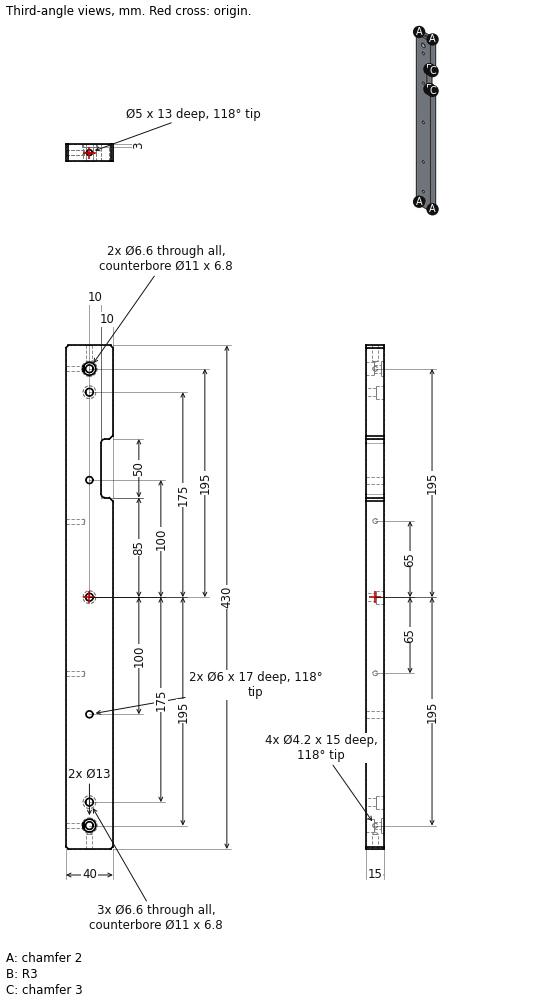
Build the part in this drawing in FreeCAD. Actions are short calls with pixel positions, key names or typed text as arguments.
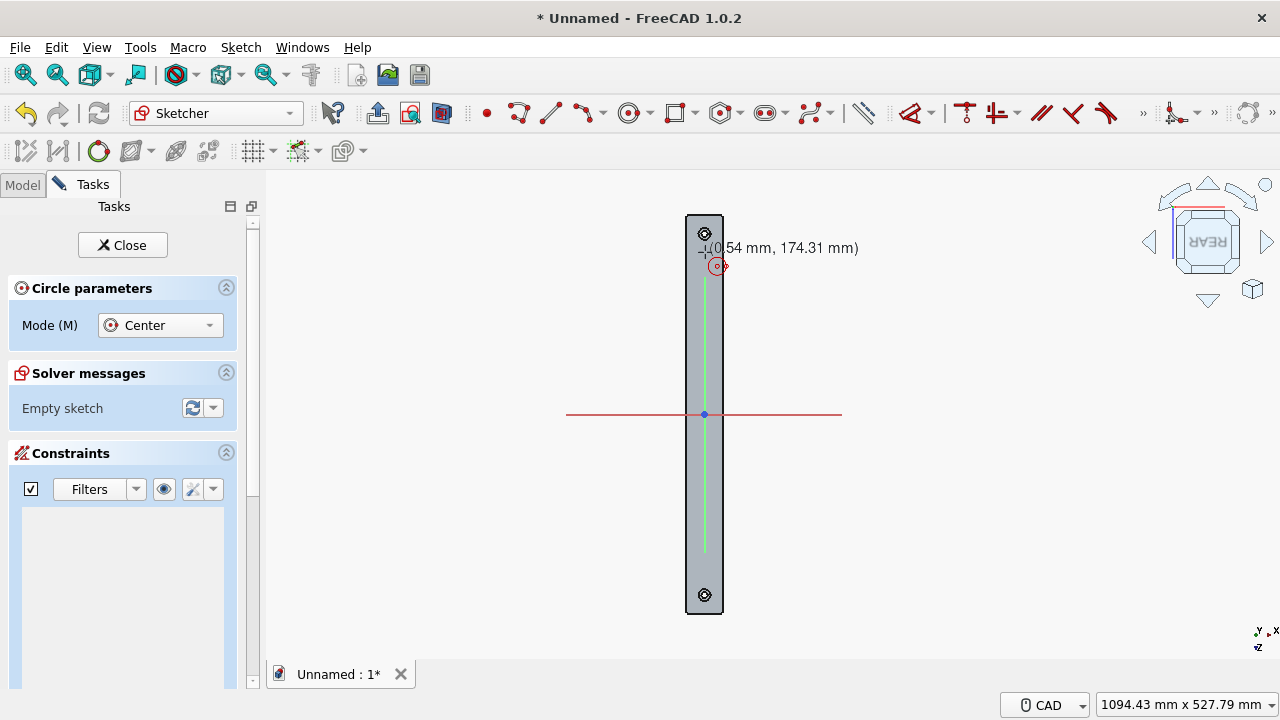
click(705, 252)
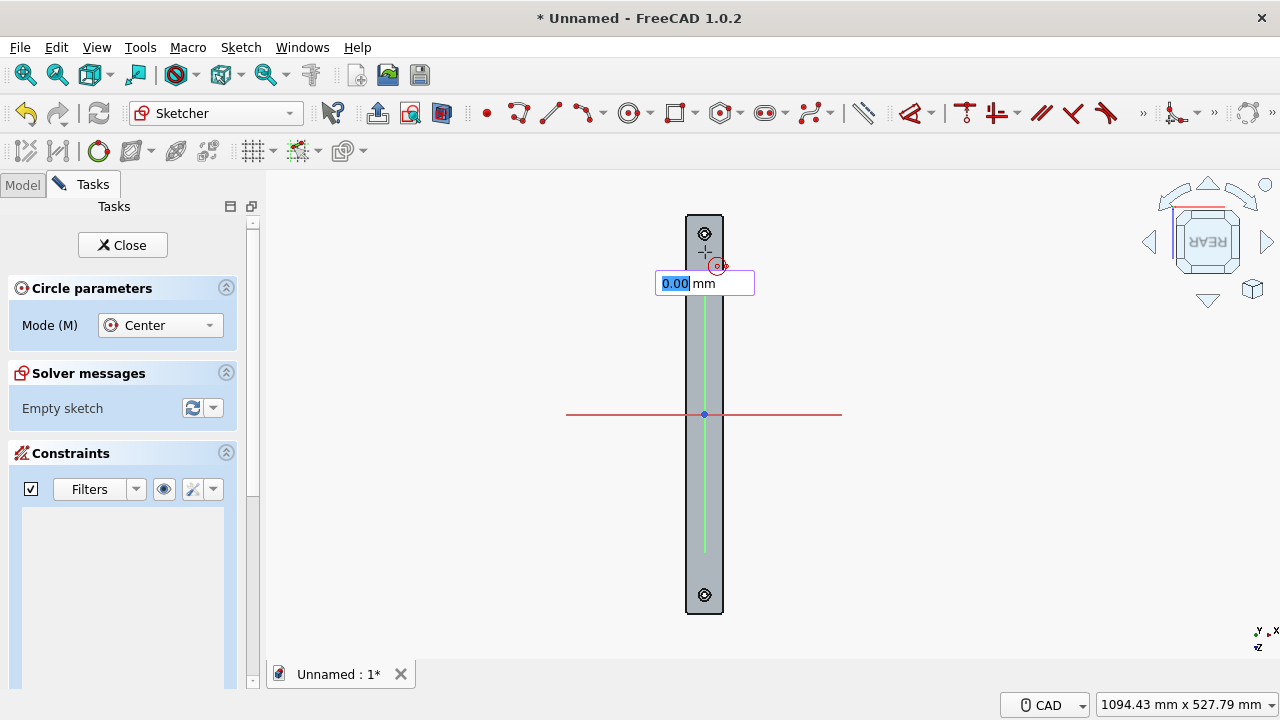
scroll(707, 251, up, 9)
move(707, 252)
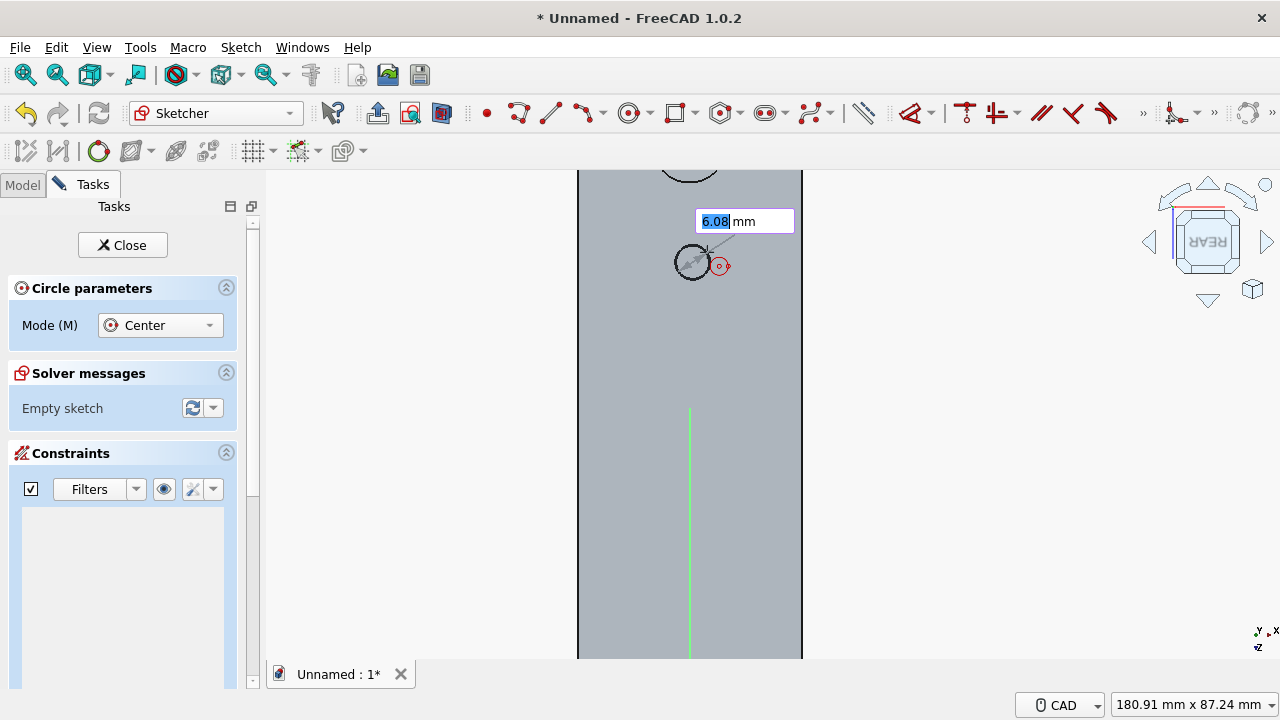
text(6.6)
key(Return)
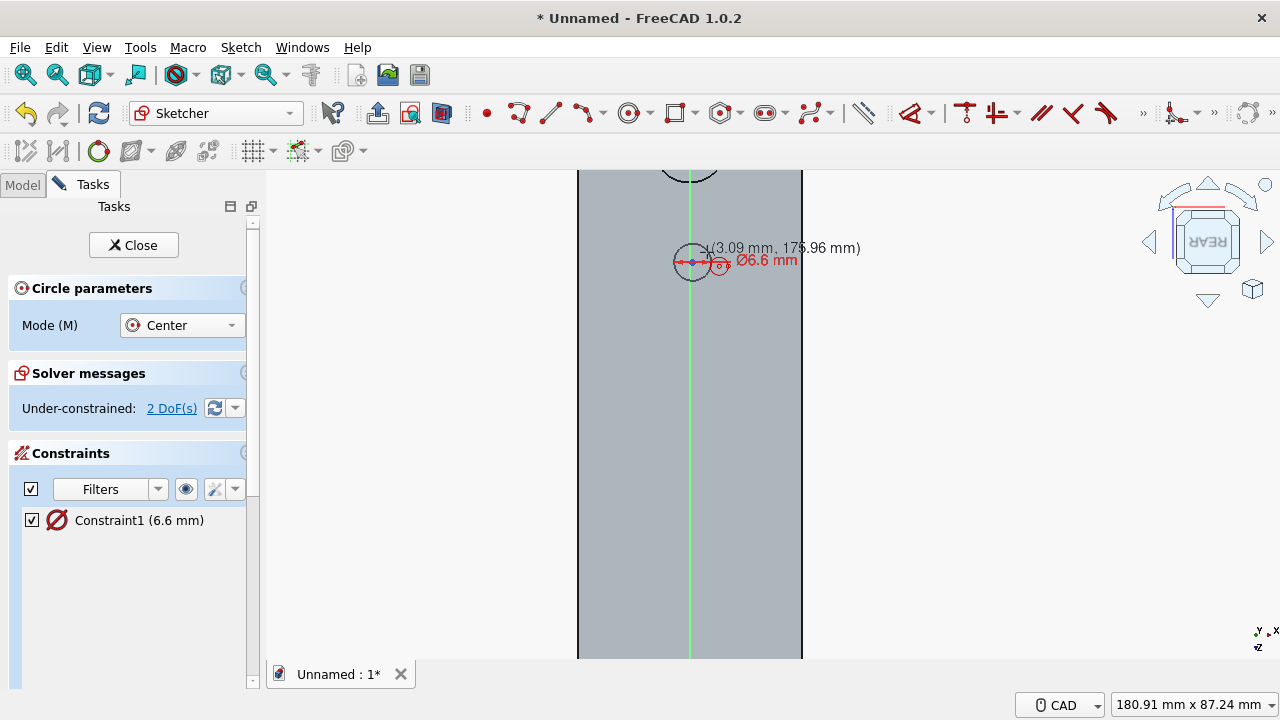
scroll(707, 251, down, 9)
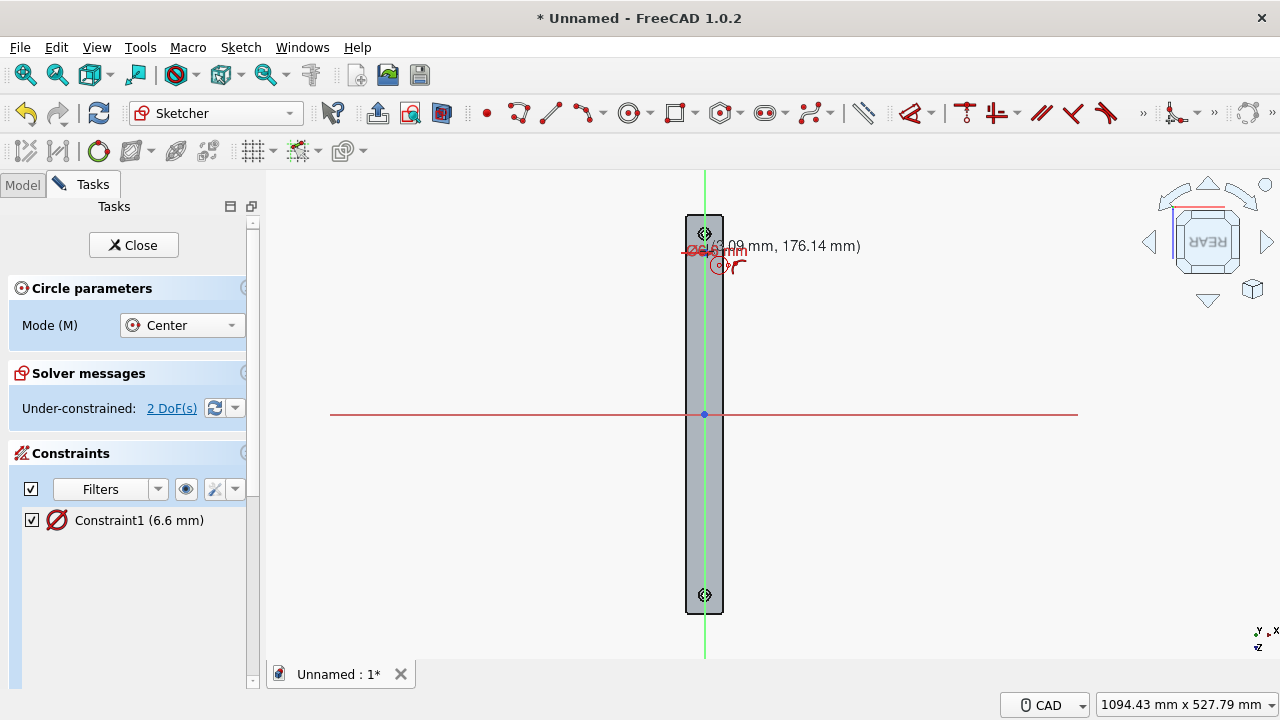
scroll(705, 577, up, 11)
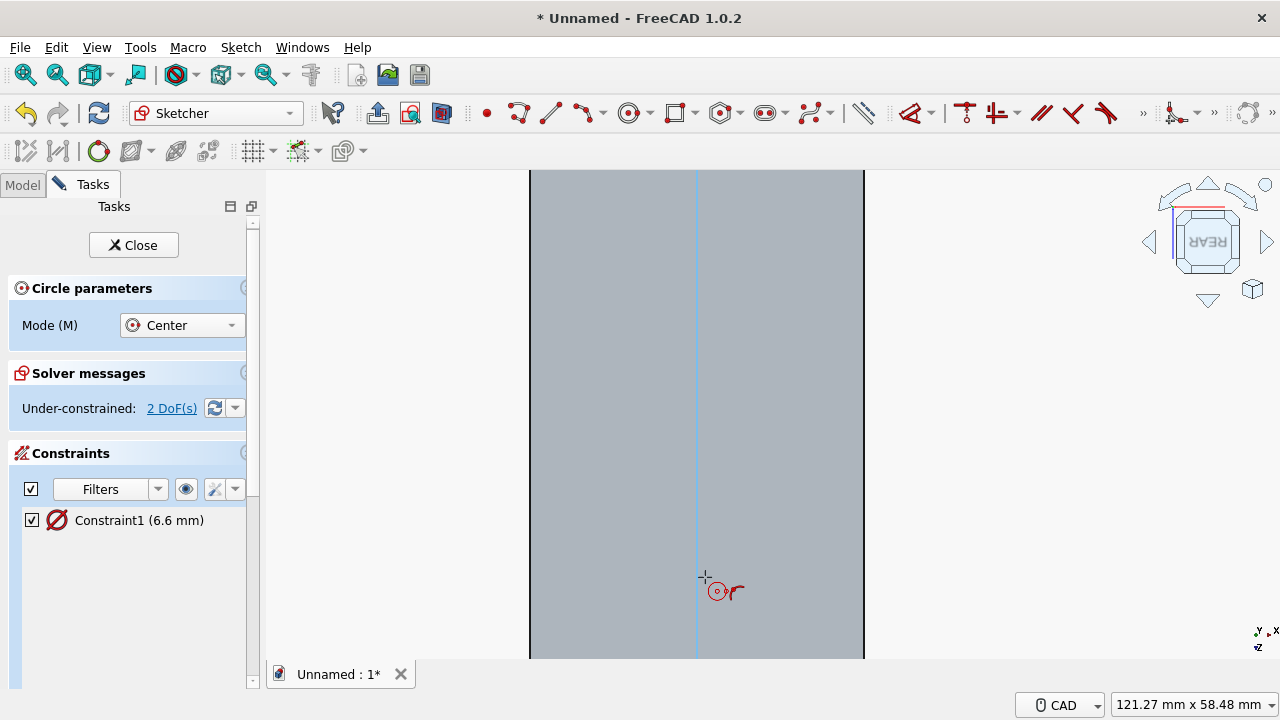
scroll(705, 578, down, 11)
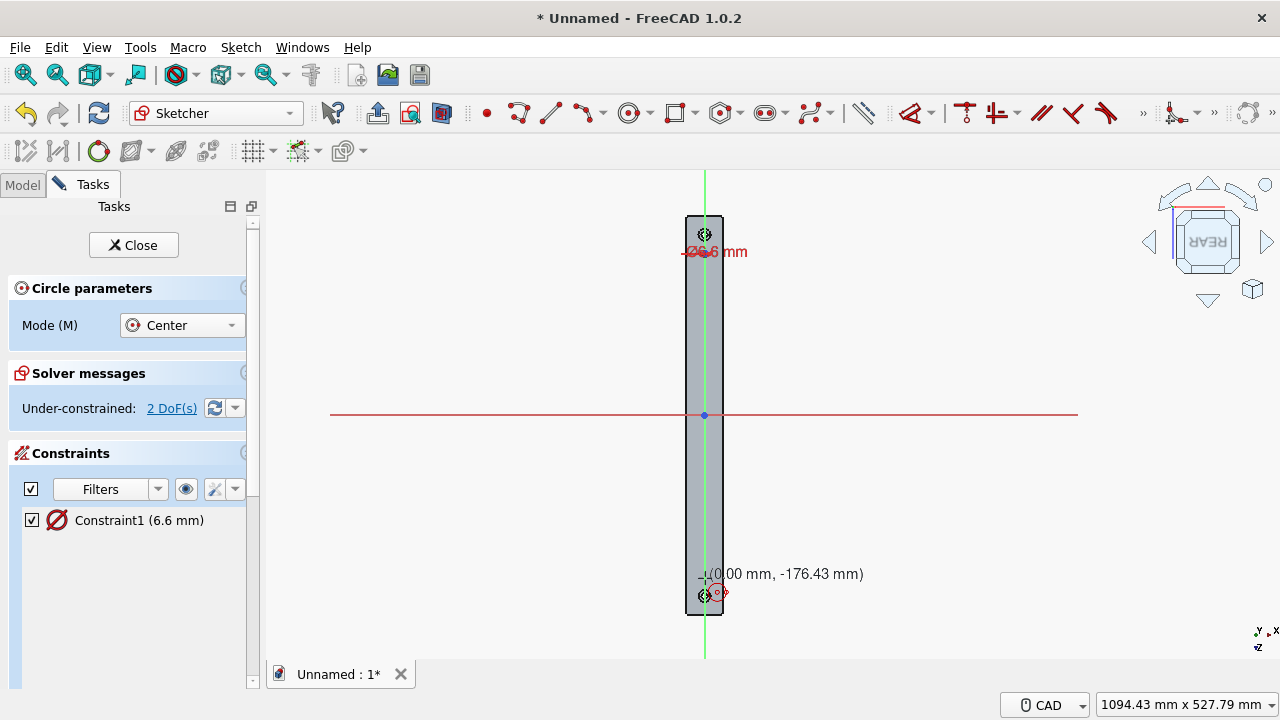
click(705, 578)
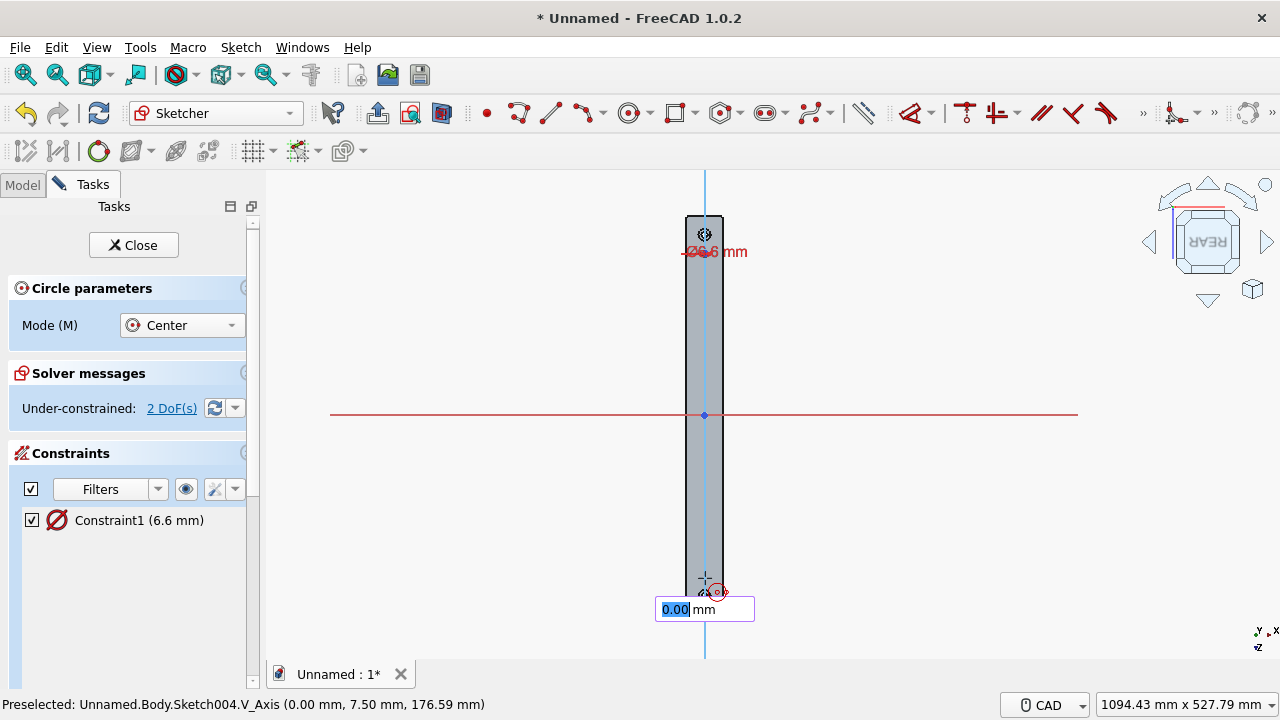
scroll(707, 576, up, 9)
move(707, 575)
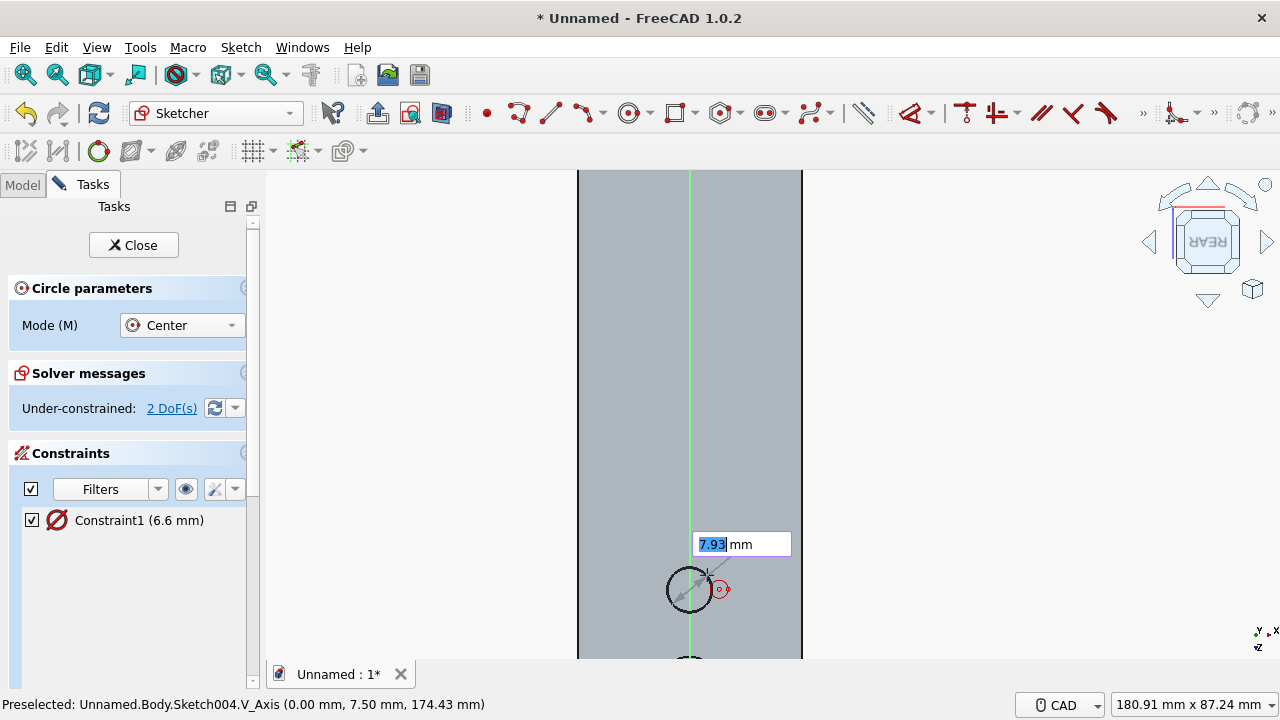
text(6.6)
key(Return)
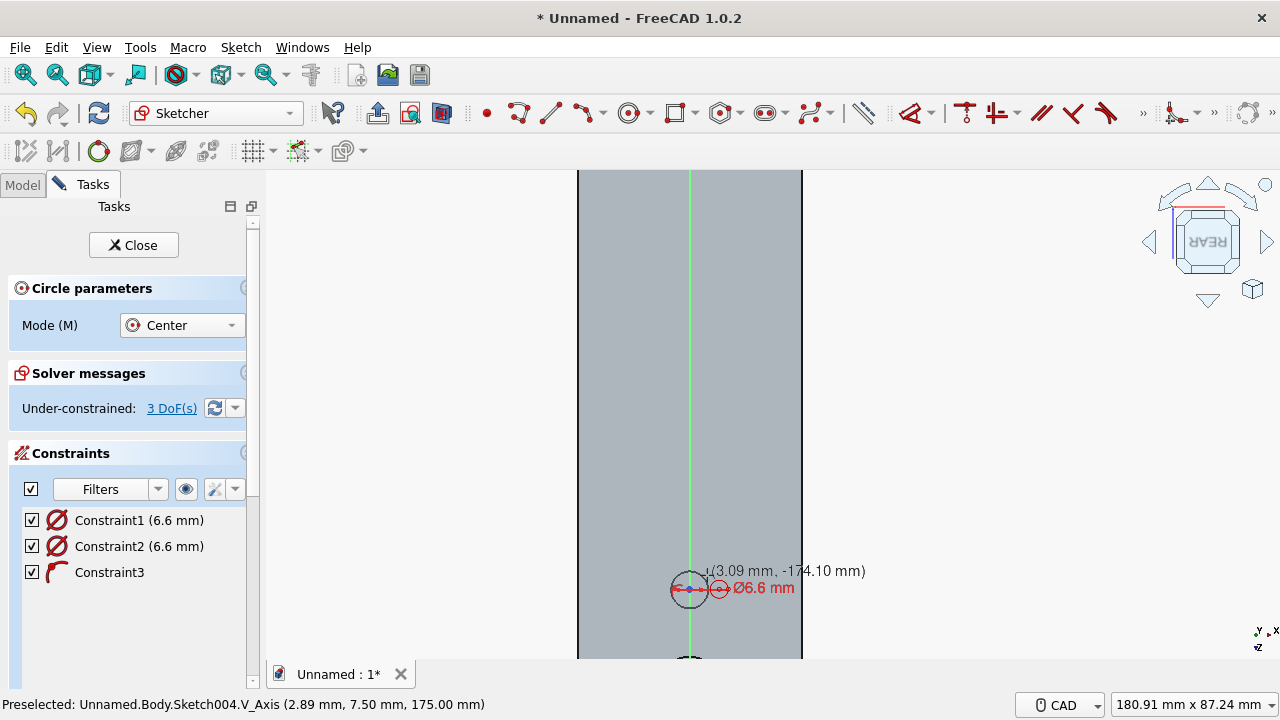
scroll(707, 576, down, 9)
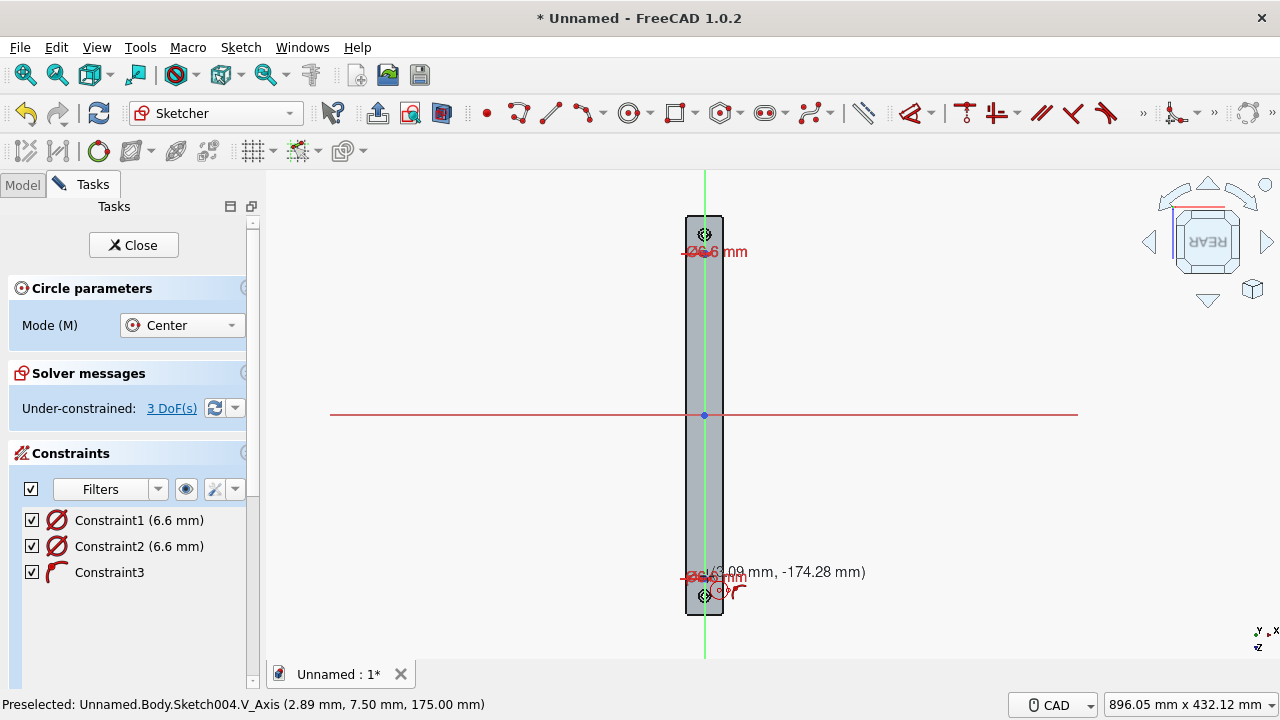
scroll(705, 415, up, 11)